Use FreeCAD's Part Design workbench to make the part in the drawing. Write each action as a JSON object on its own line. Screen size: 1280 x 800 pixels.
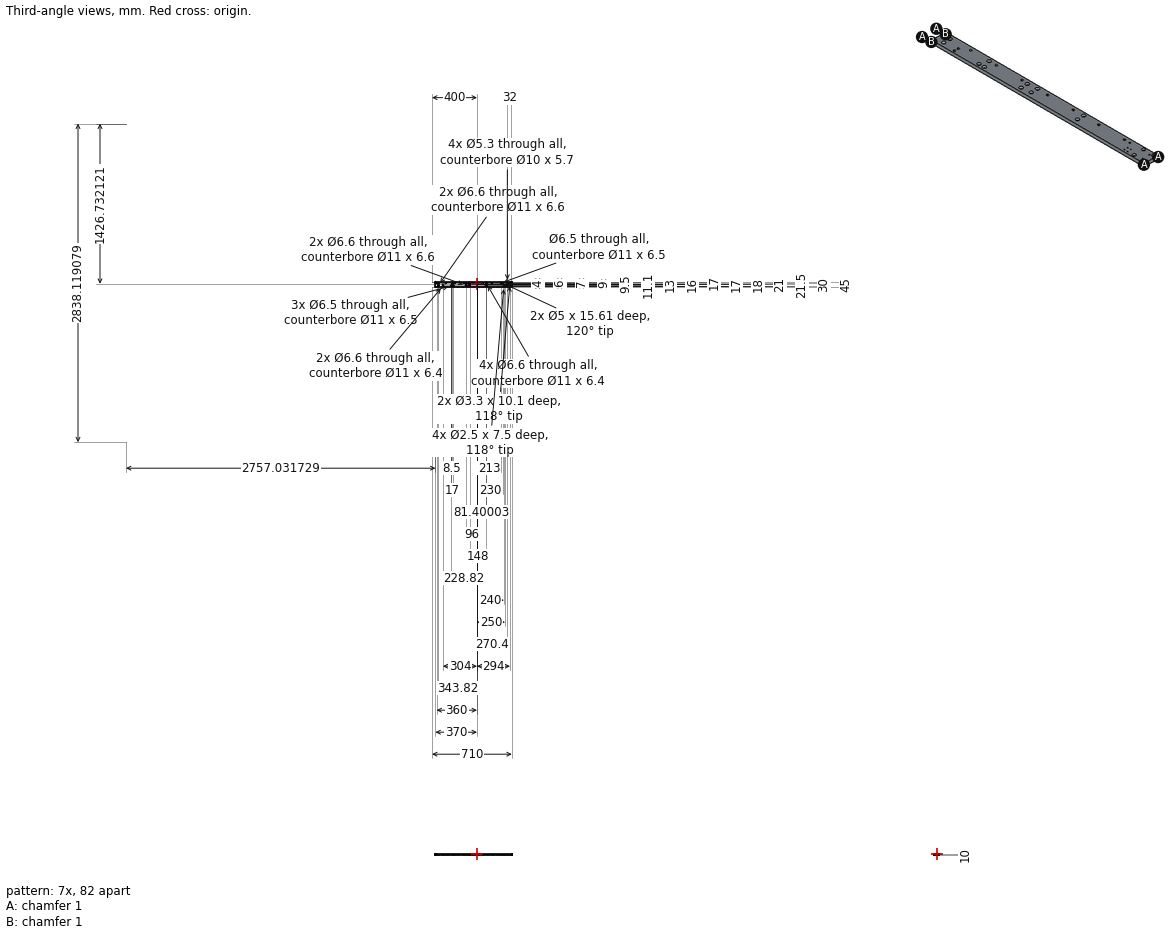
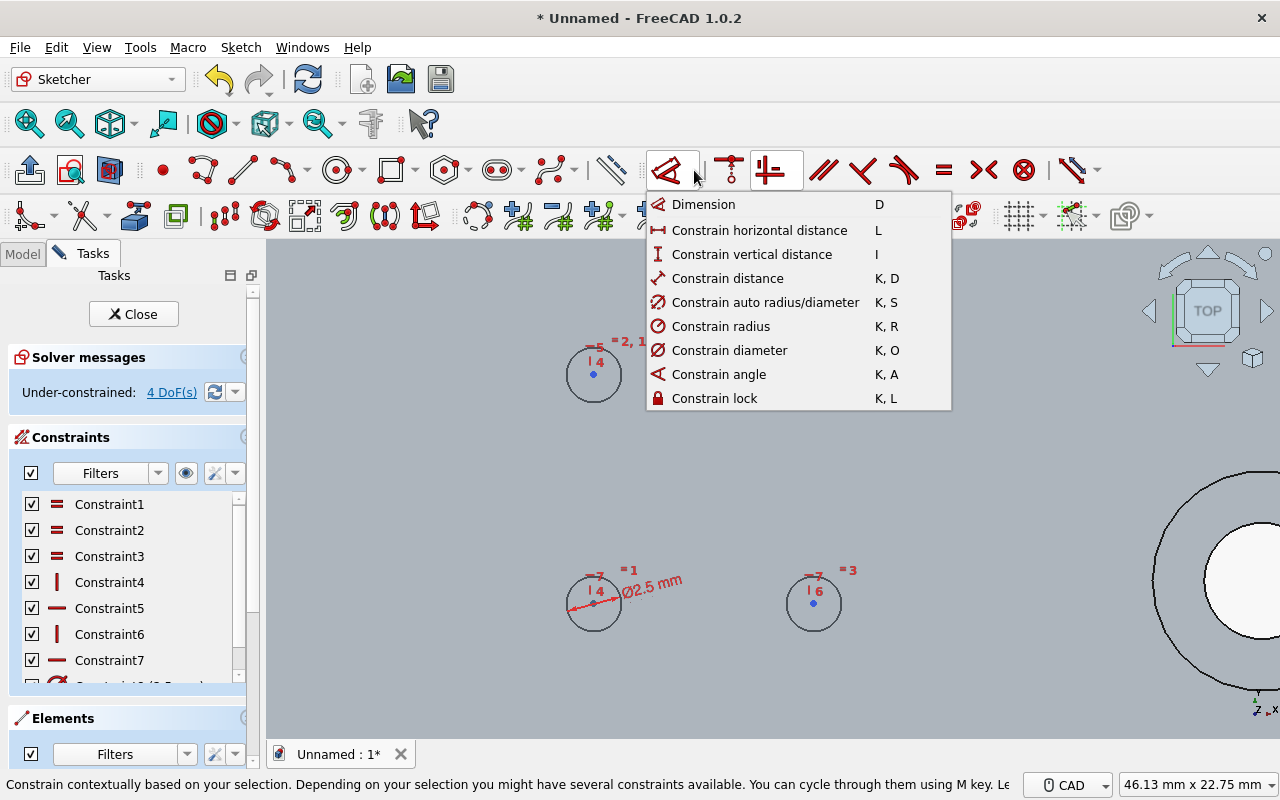
{"action": "left_click", "coordinate": [799, 230]}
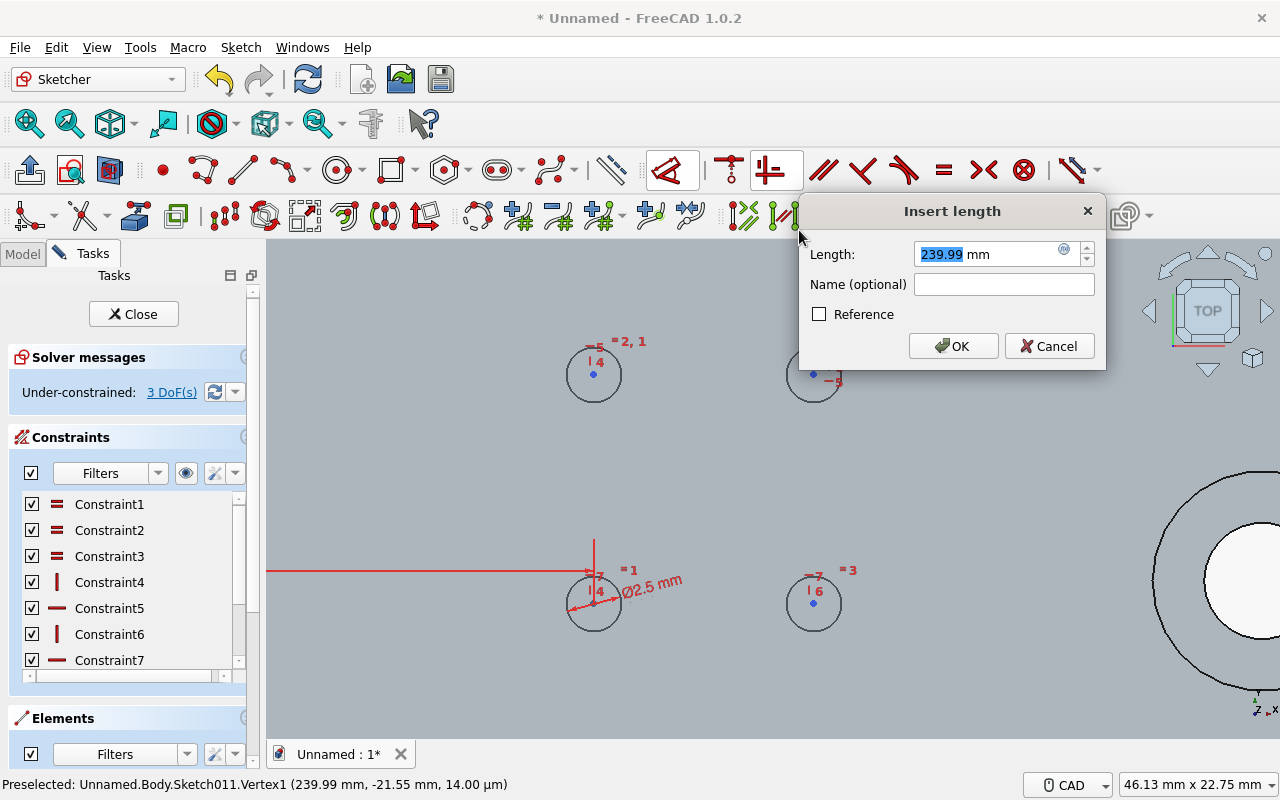
{"action": "type", "text": "240"}
{"action": "key", "text": "Return"}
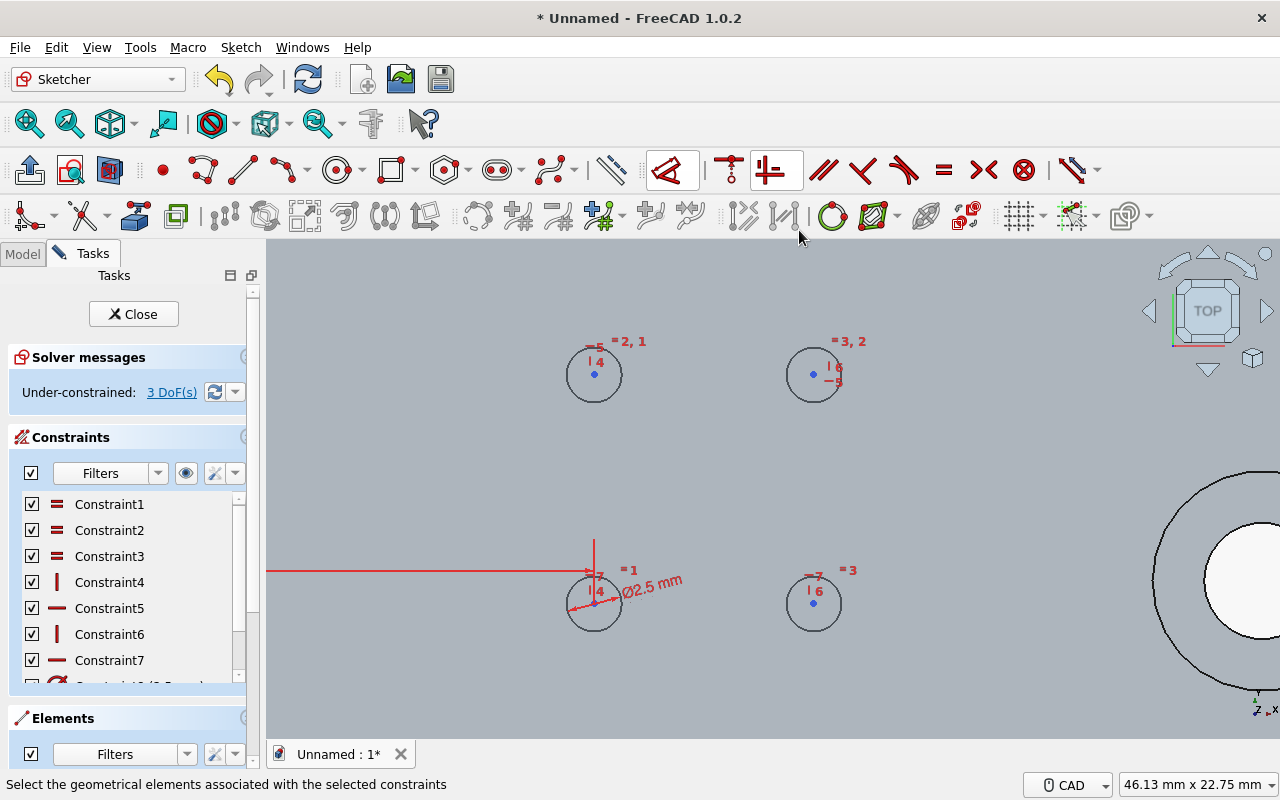
{"action": "left_click", "coordinate": [814, 375]}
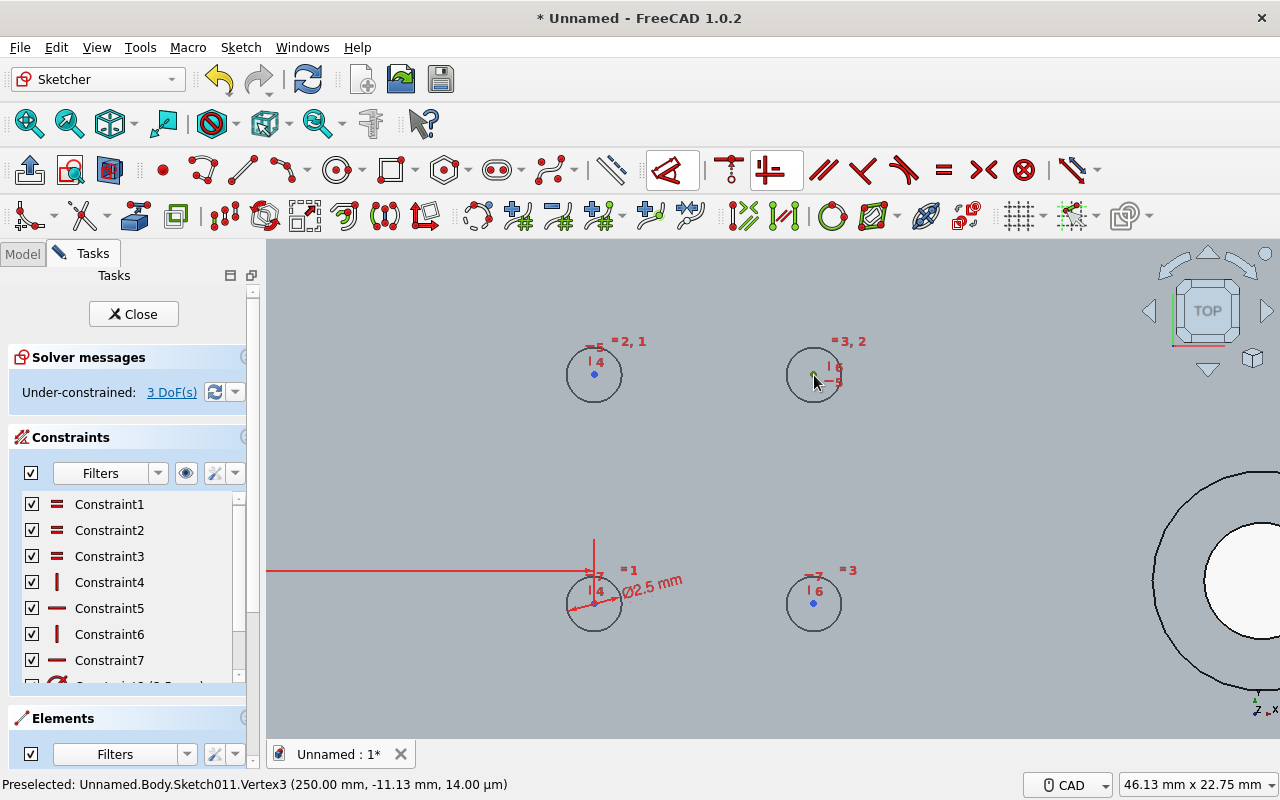
{"action": "key", "text": "l"}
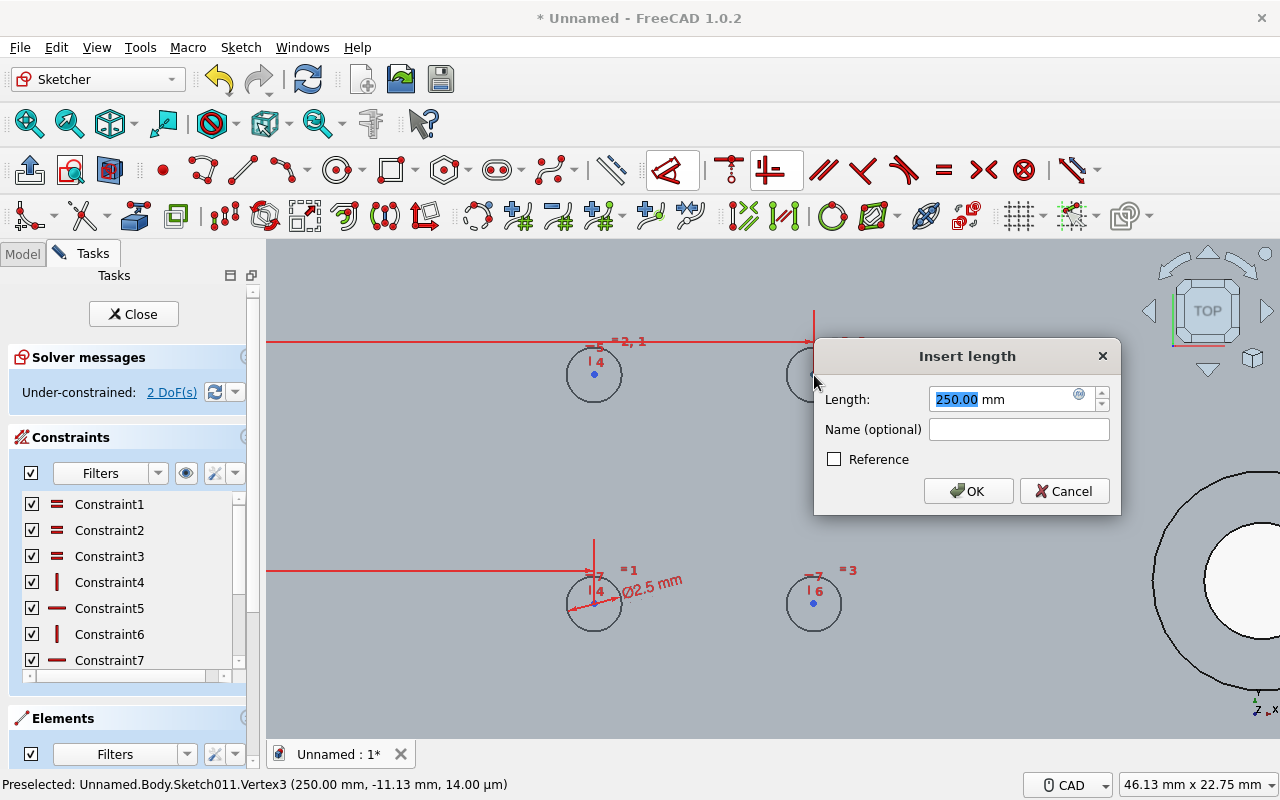
{"action": "type", "text": "250"}
{"action": "key", "text": "Return"}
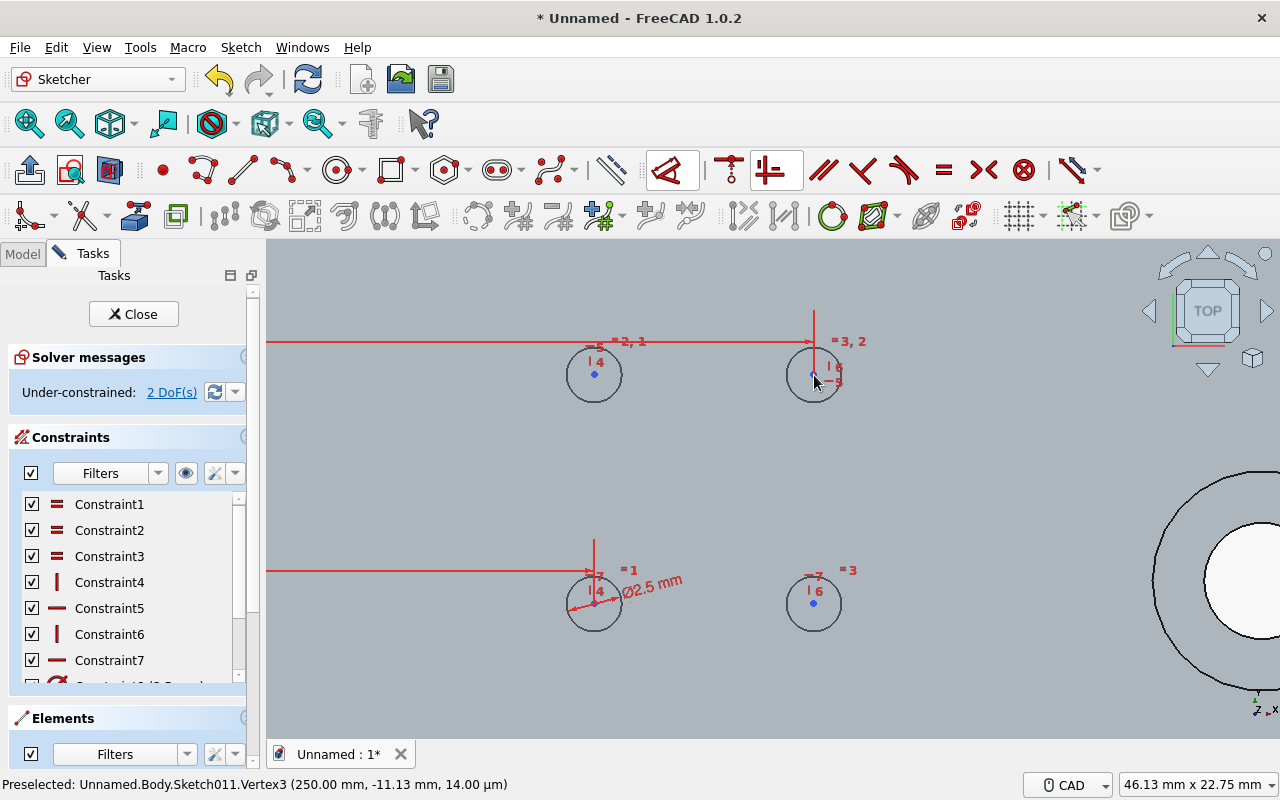
{"action": "left_click", "coordinate": [594, 604]}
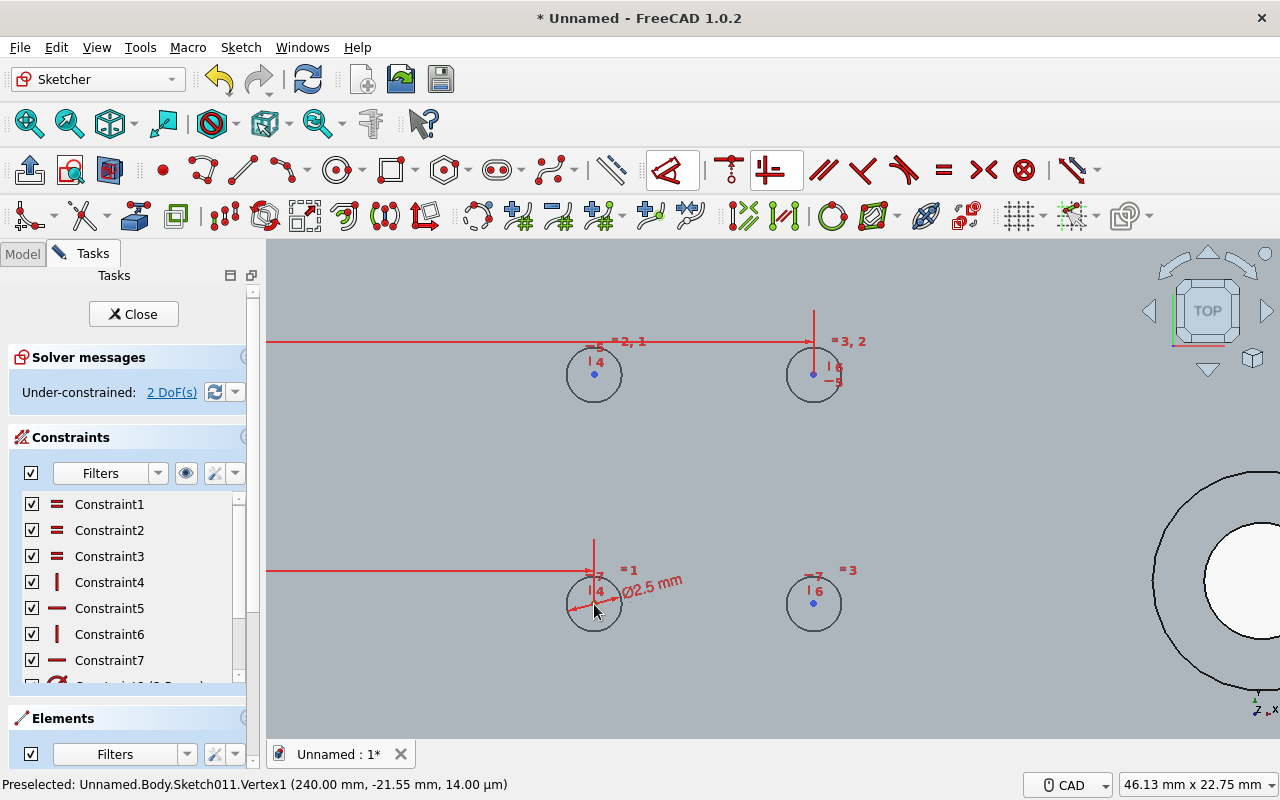
{"action": "left_click", "coordinate": [694, 170]}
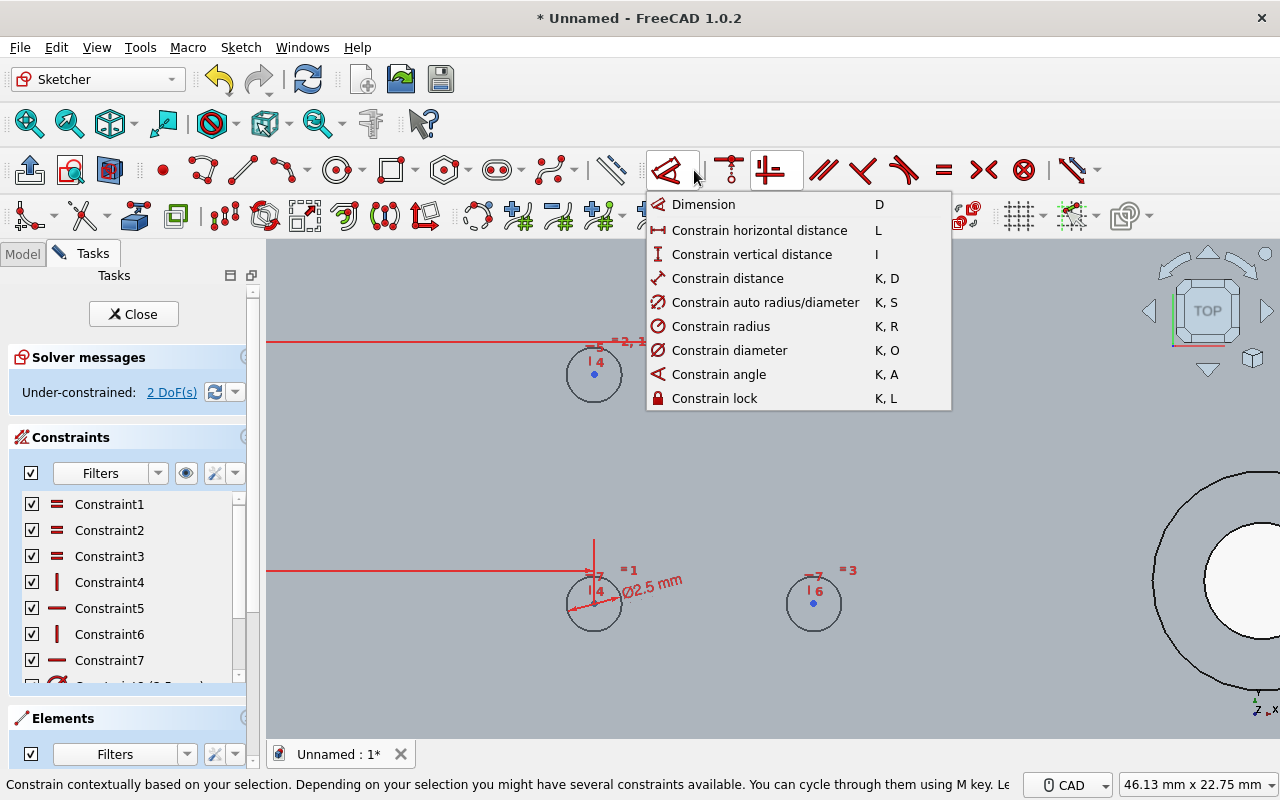
{"action": "left_click", "coordinate": [799, 254]}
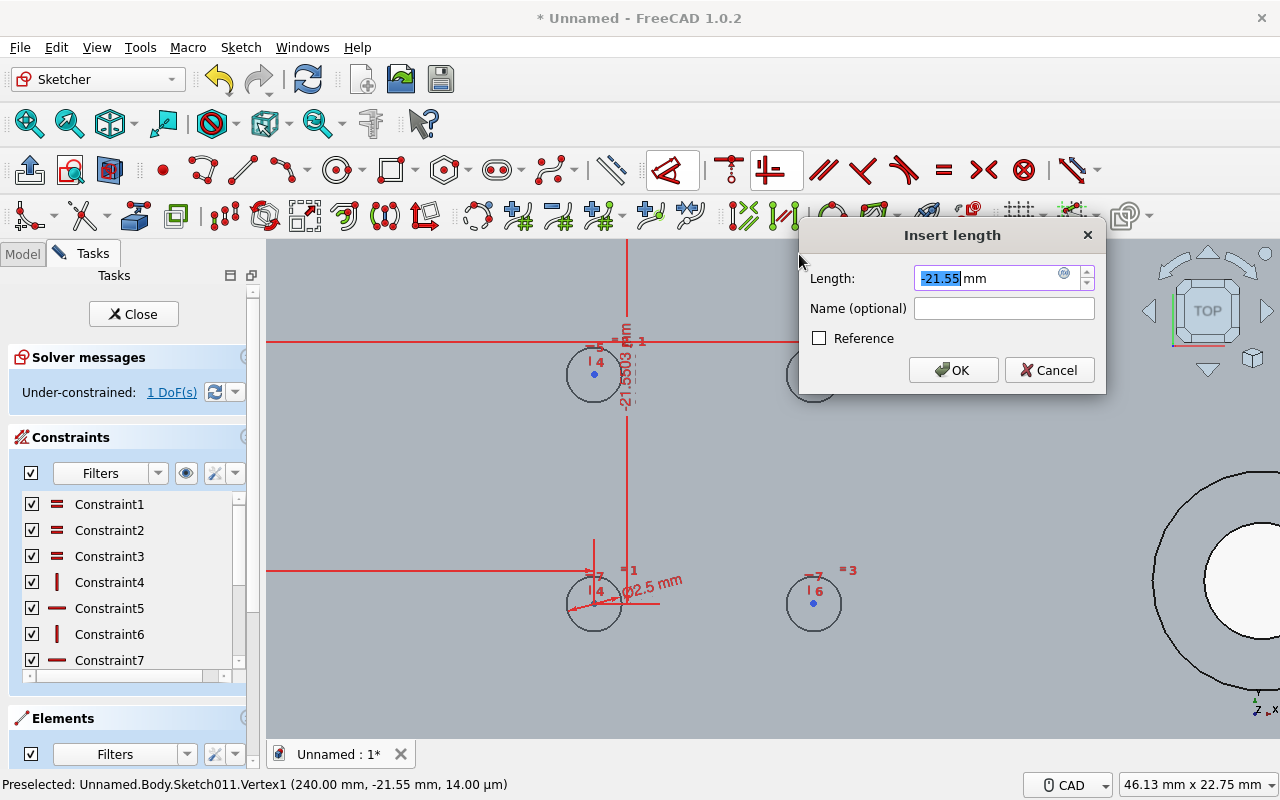
{"action": "type", "text": "-21.5"}
{"action": "key", "text": "Return"}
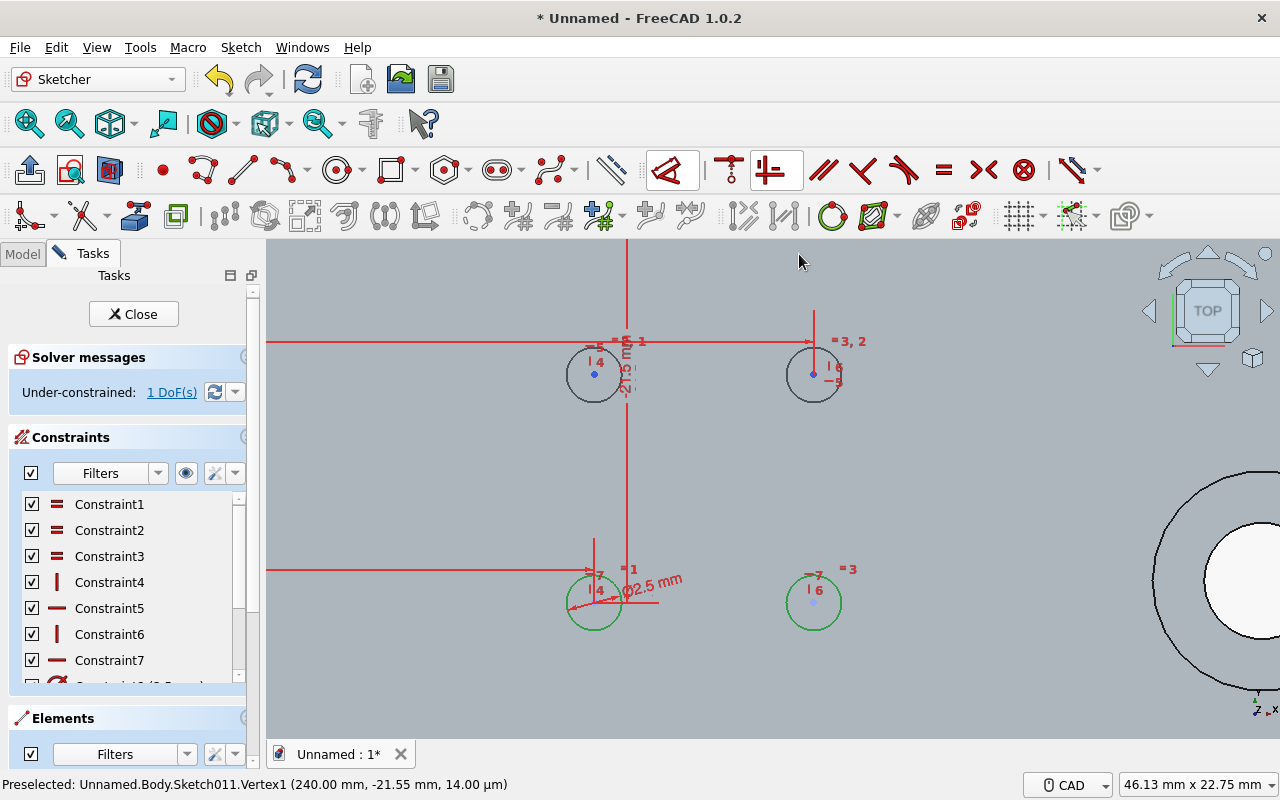
{"action": "left_click", "coordinate": [594, 375]}